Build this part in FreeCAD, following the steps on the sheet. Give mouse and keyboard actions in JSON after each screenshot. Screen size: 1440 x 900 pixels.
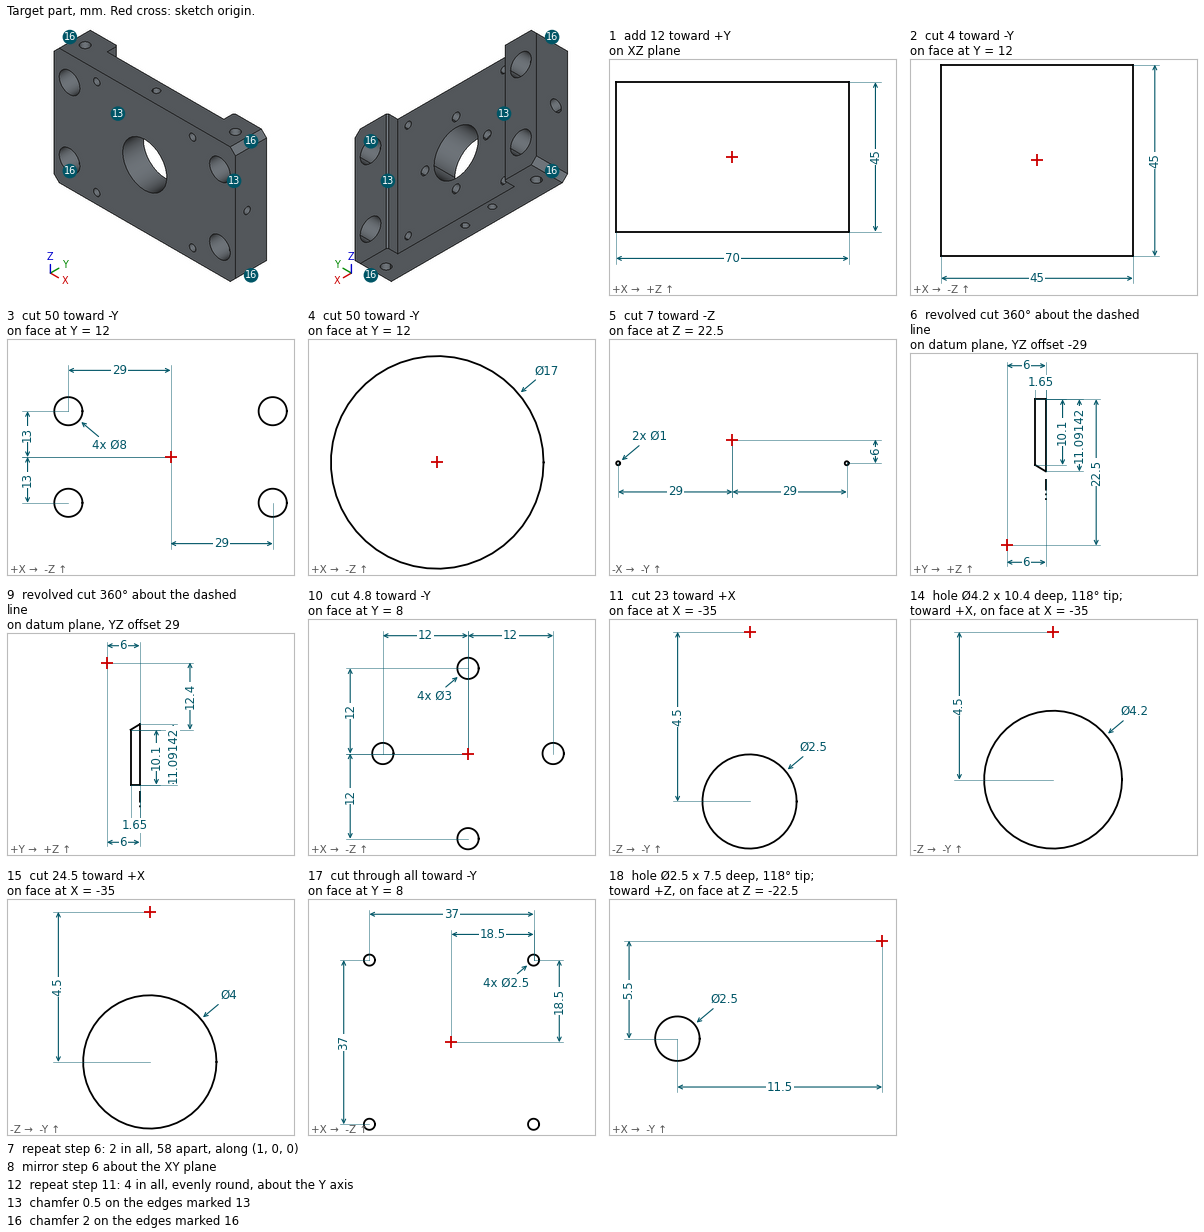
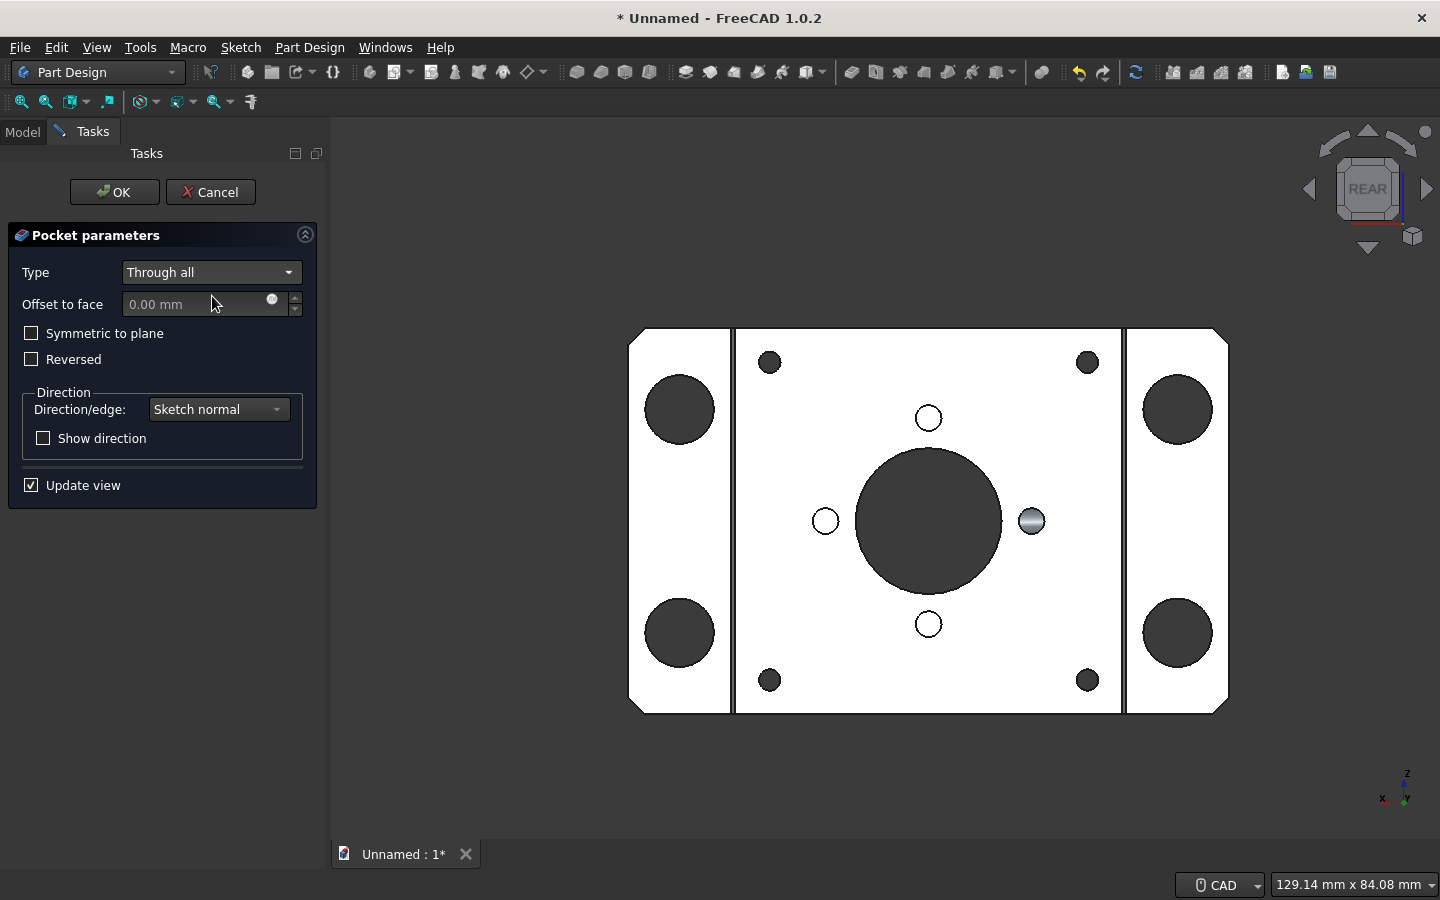
{"action": "left_click", "coordinate": [115, 192]}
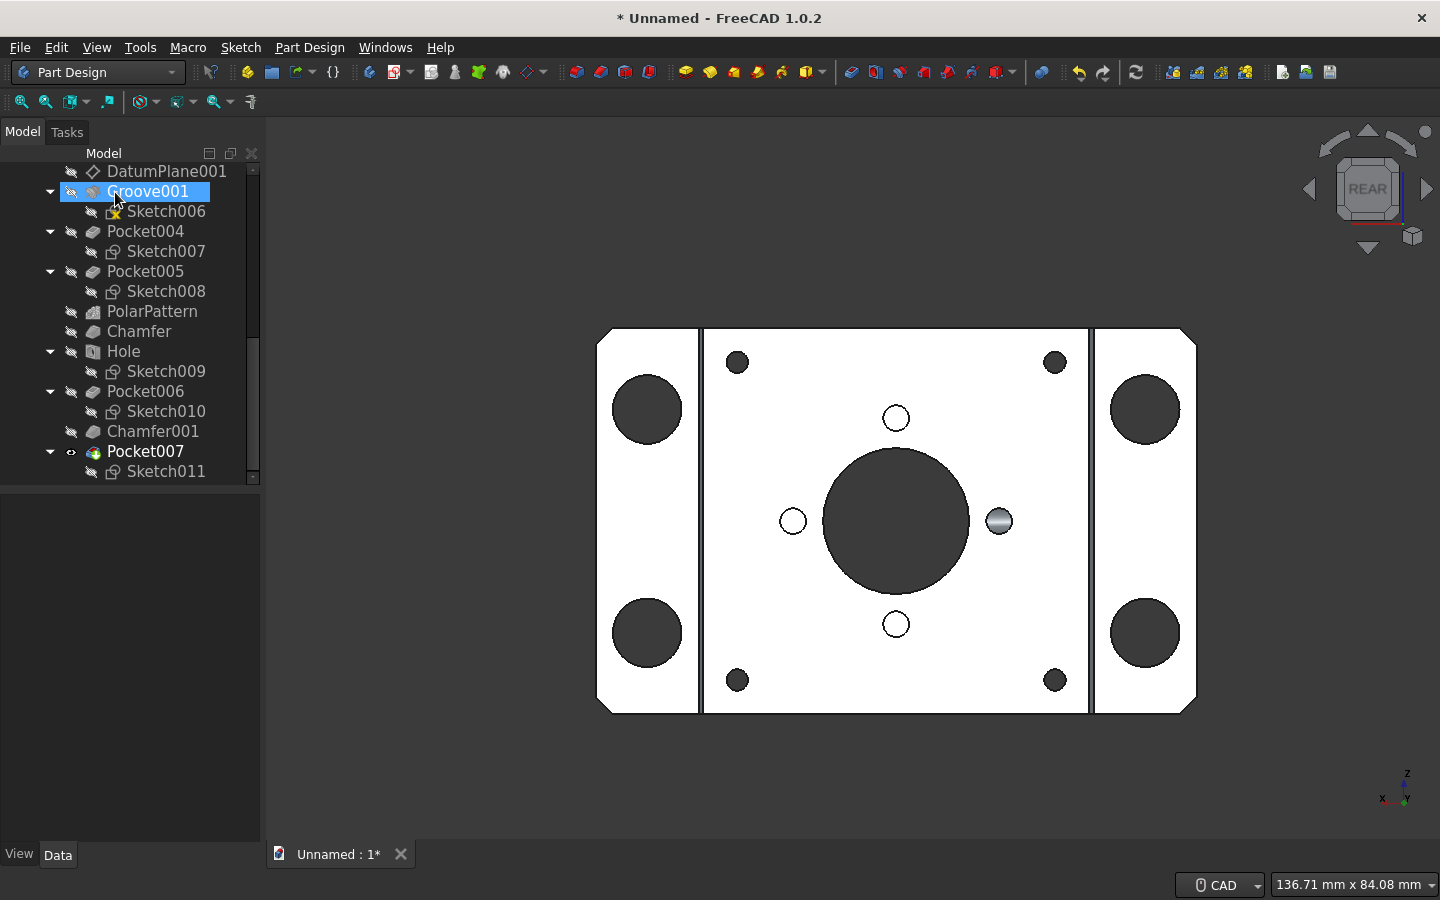
{"action": "key", "text": "5"}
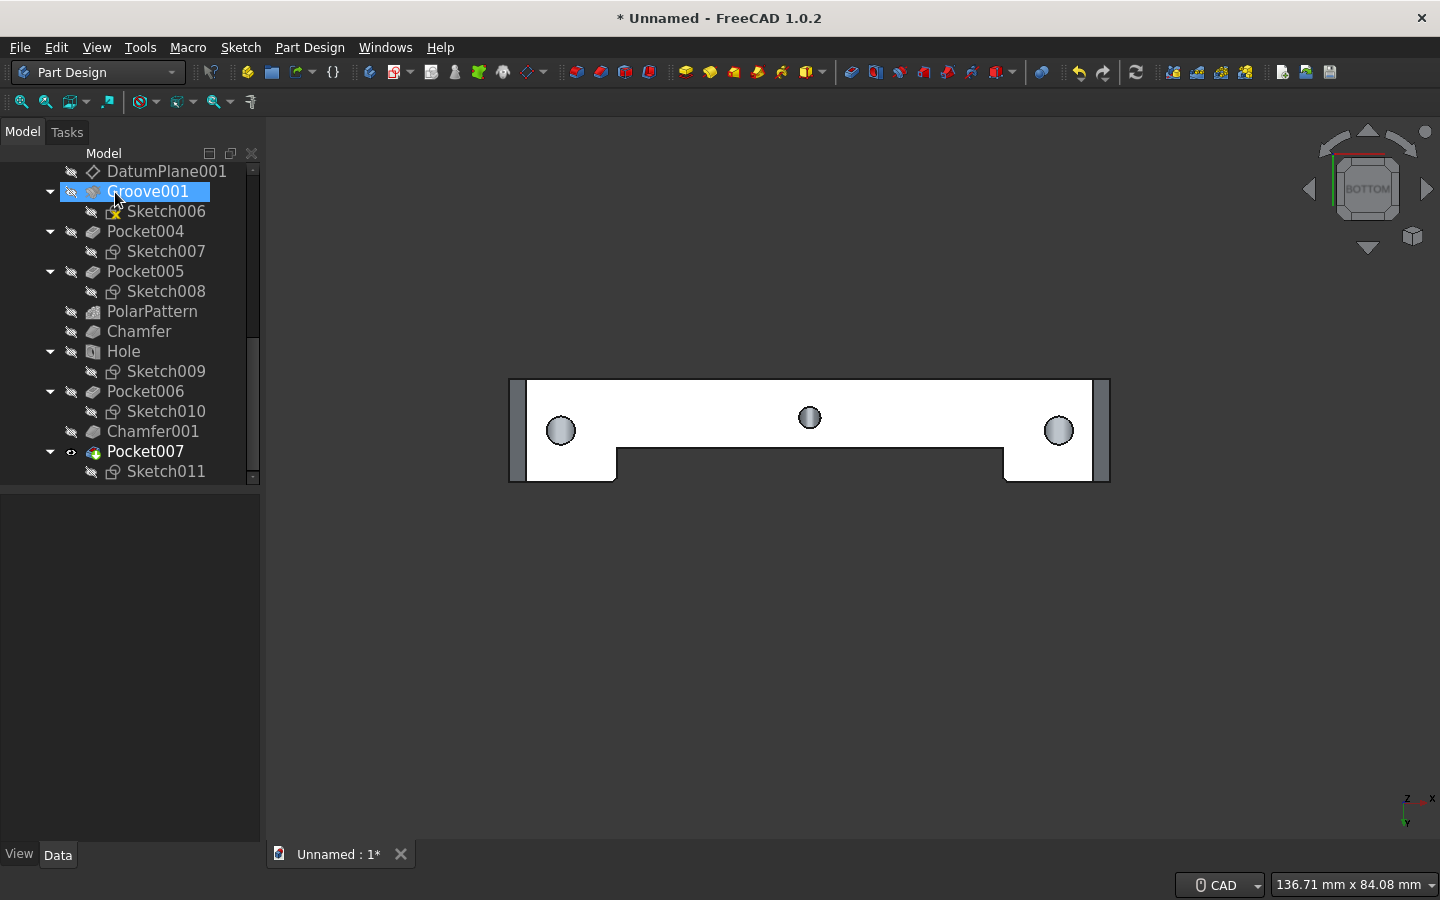
{"action": "left_click", "coordinate": [972, 415]}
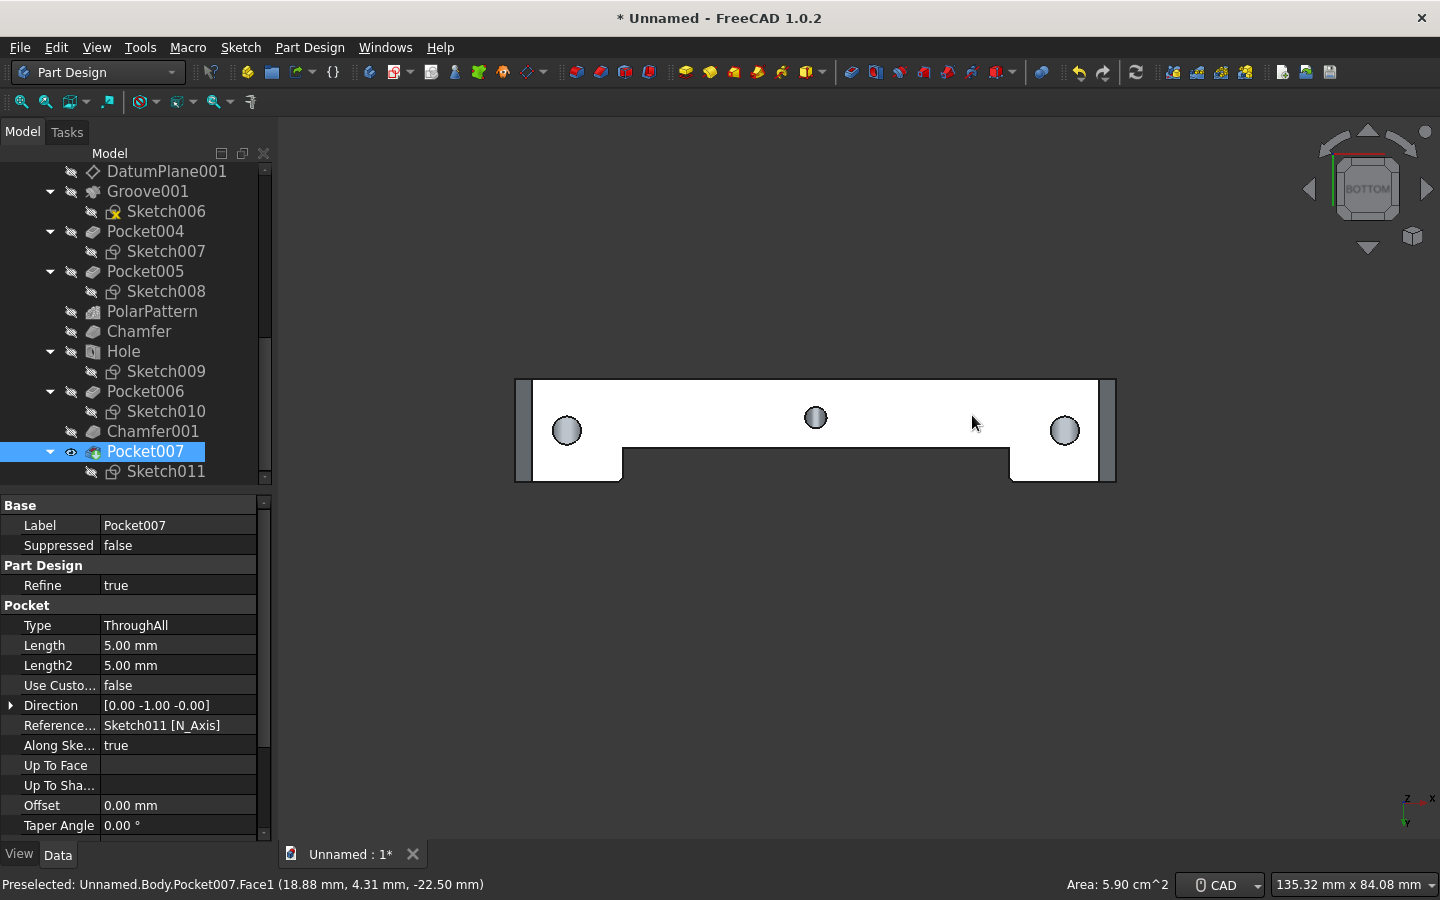
{"action": "left_click", "coordinate": [394, 72]}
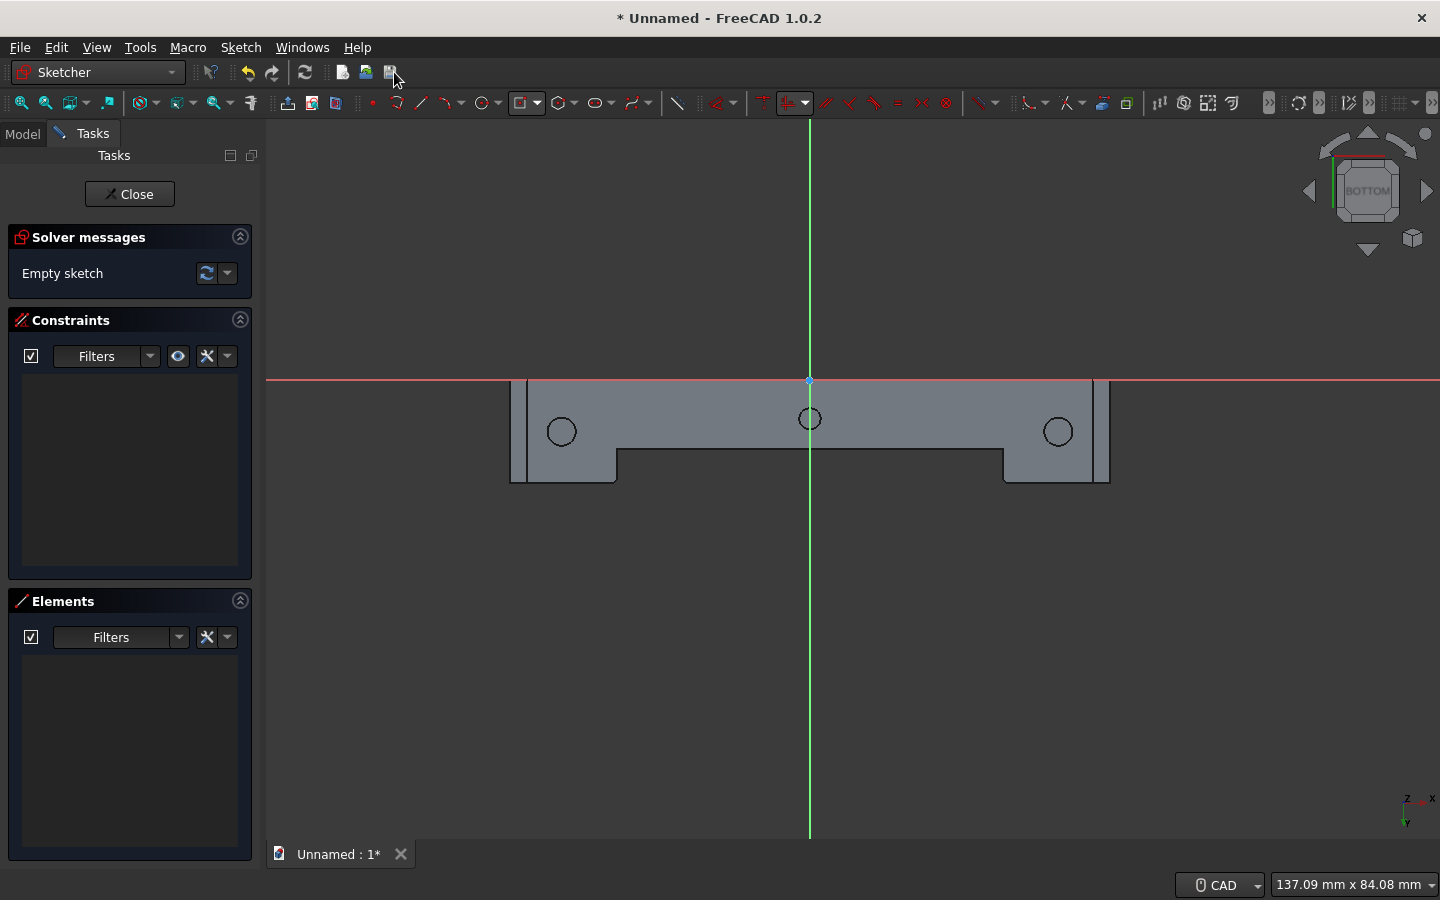
{"action": "scroll", "coordinate": [708, 425], "scroll_direction": "up", "scroll_amount": 15}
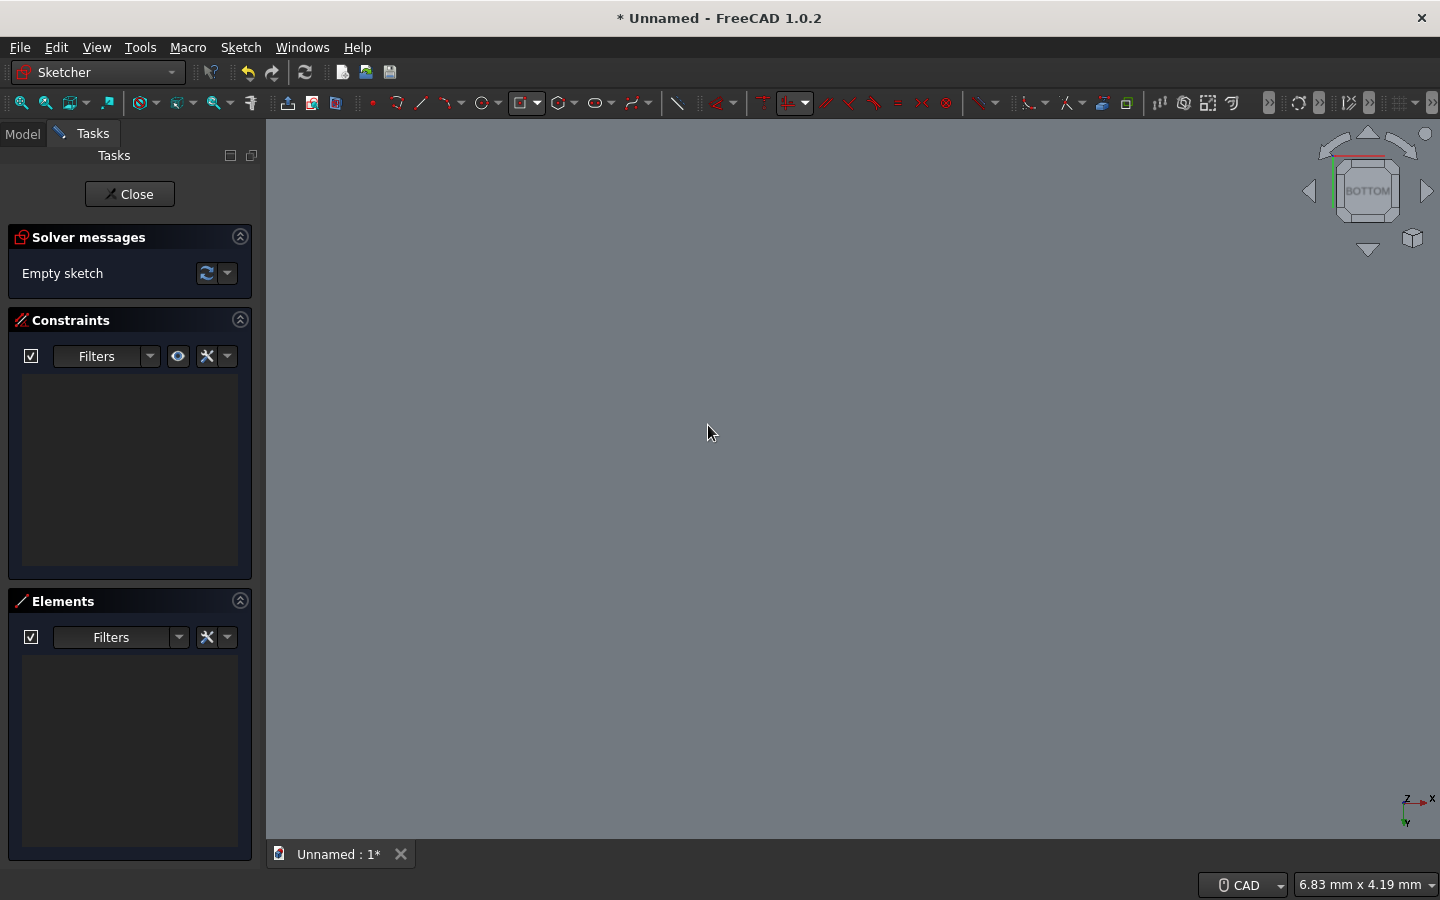
{"action": "left_click", "coordinate": [482, 104]}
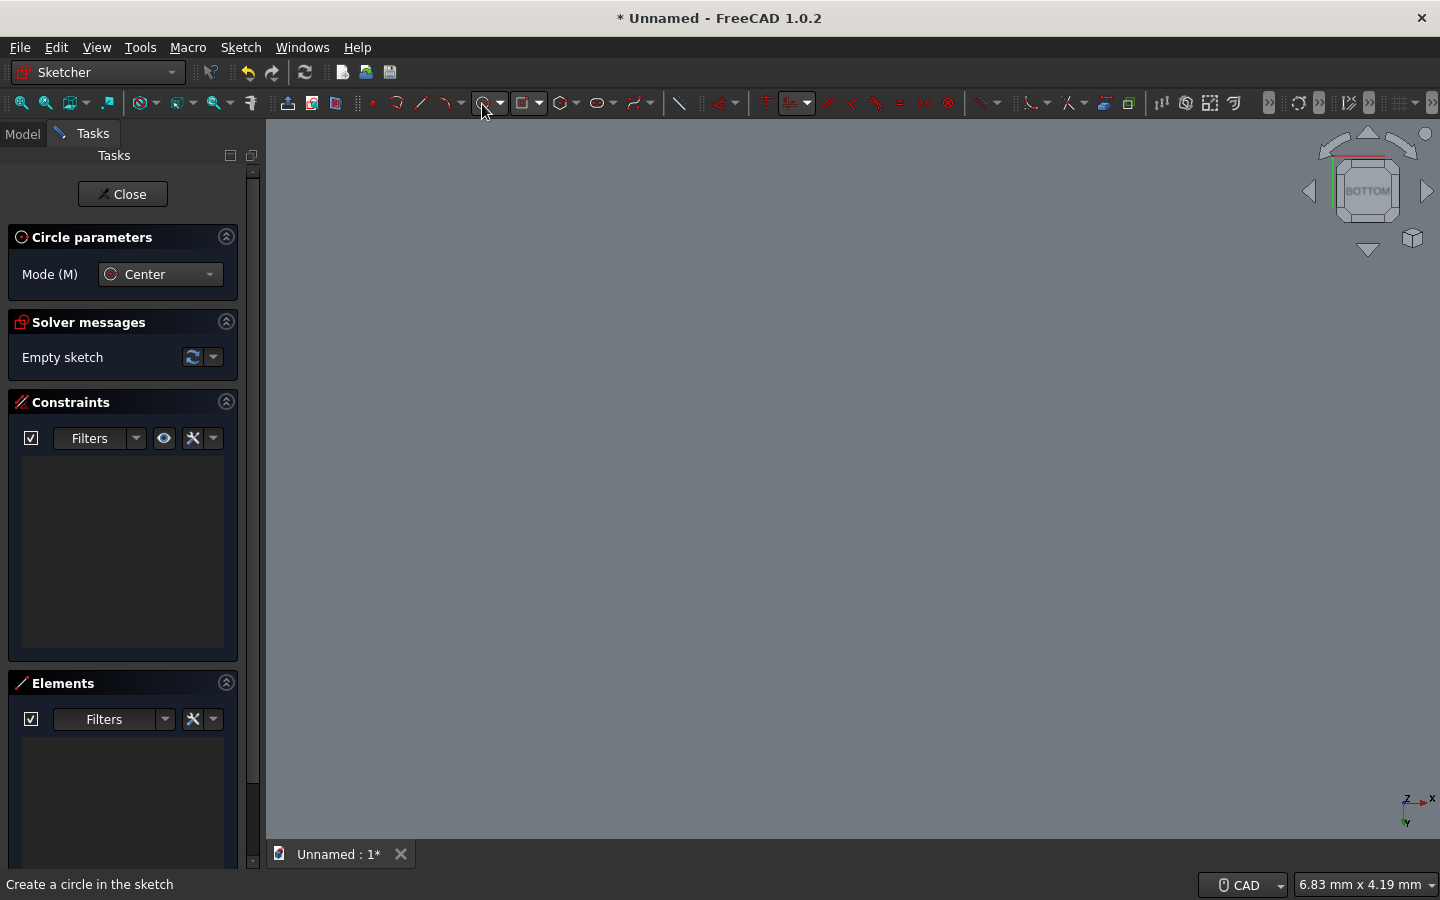
{"action": "left_click", "coordinate": [771, 465]}
{"action": "mouse_move", "coordinate": [923, 313]}